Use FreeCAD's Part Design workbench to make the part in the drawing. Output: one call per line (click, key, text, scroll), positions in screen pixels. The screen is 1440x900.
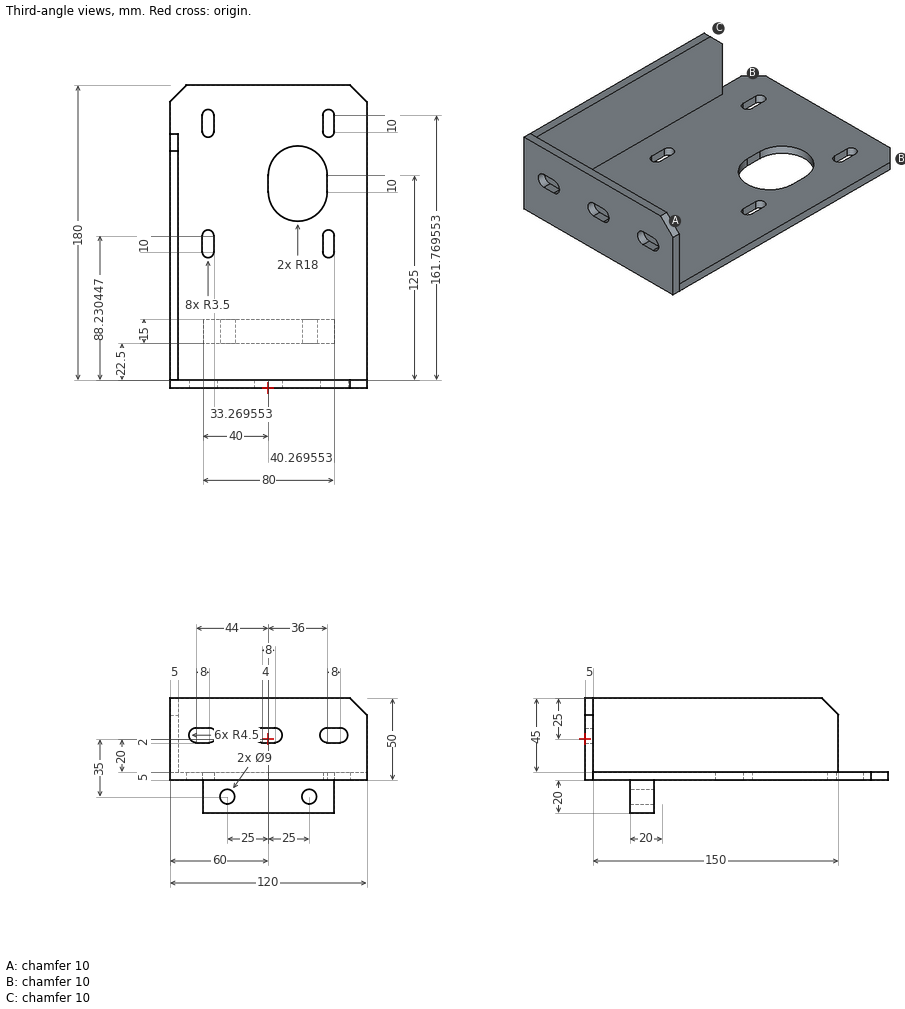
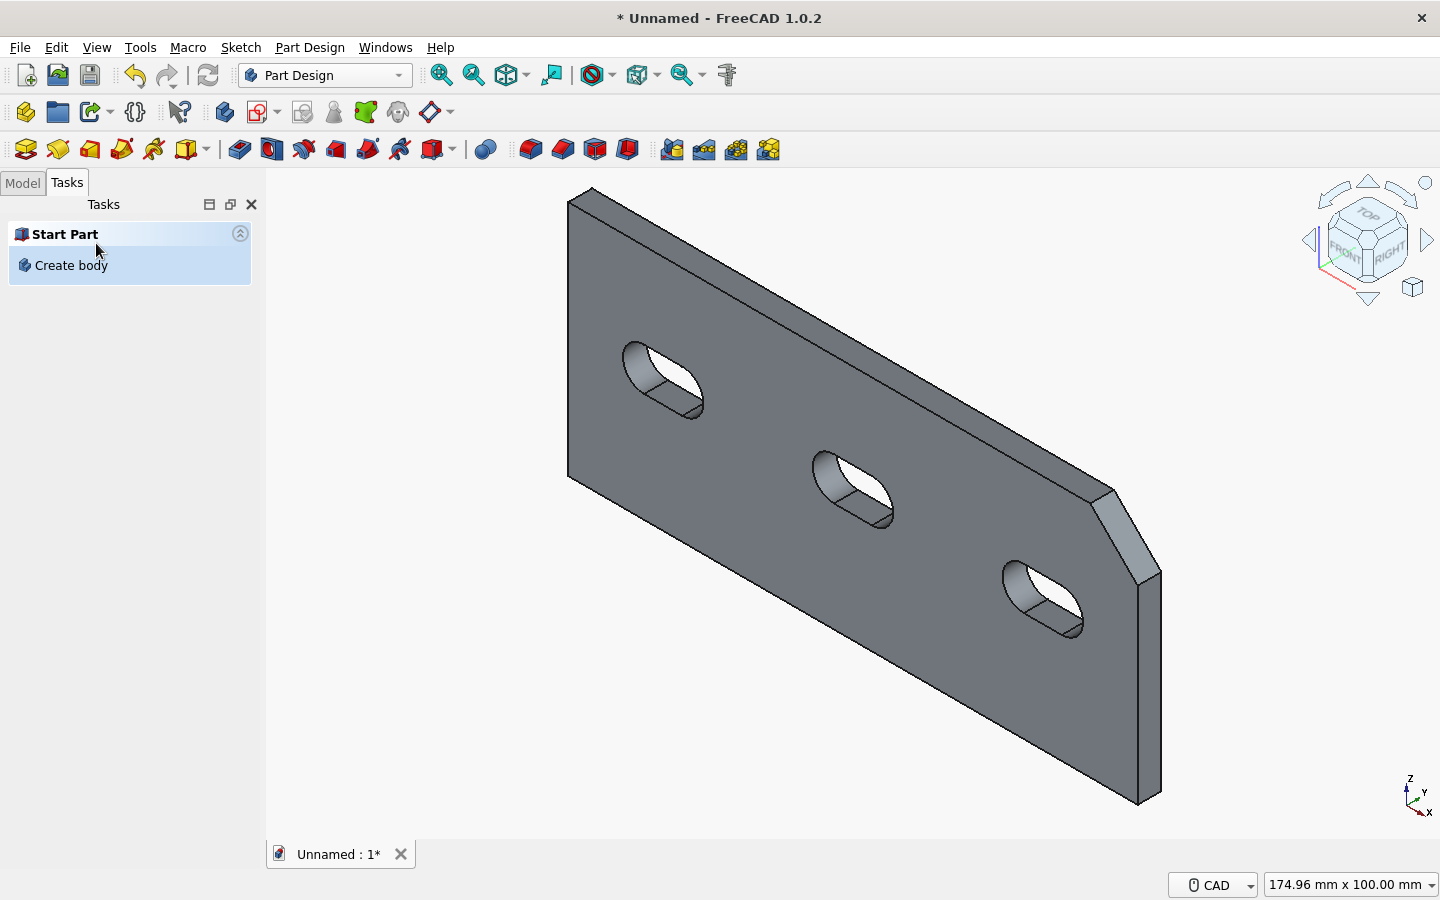
click(226, 112)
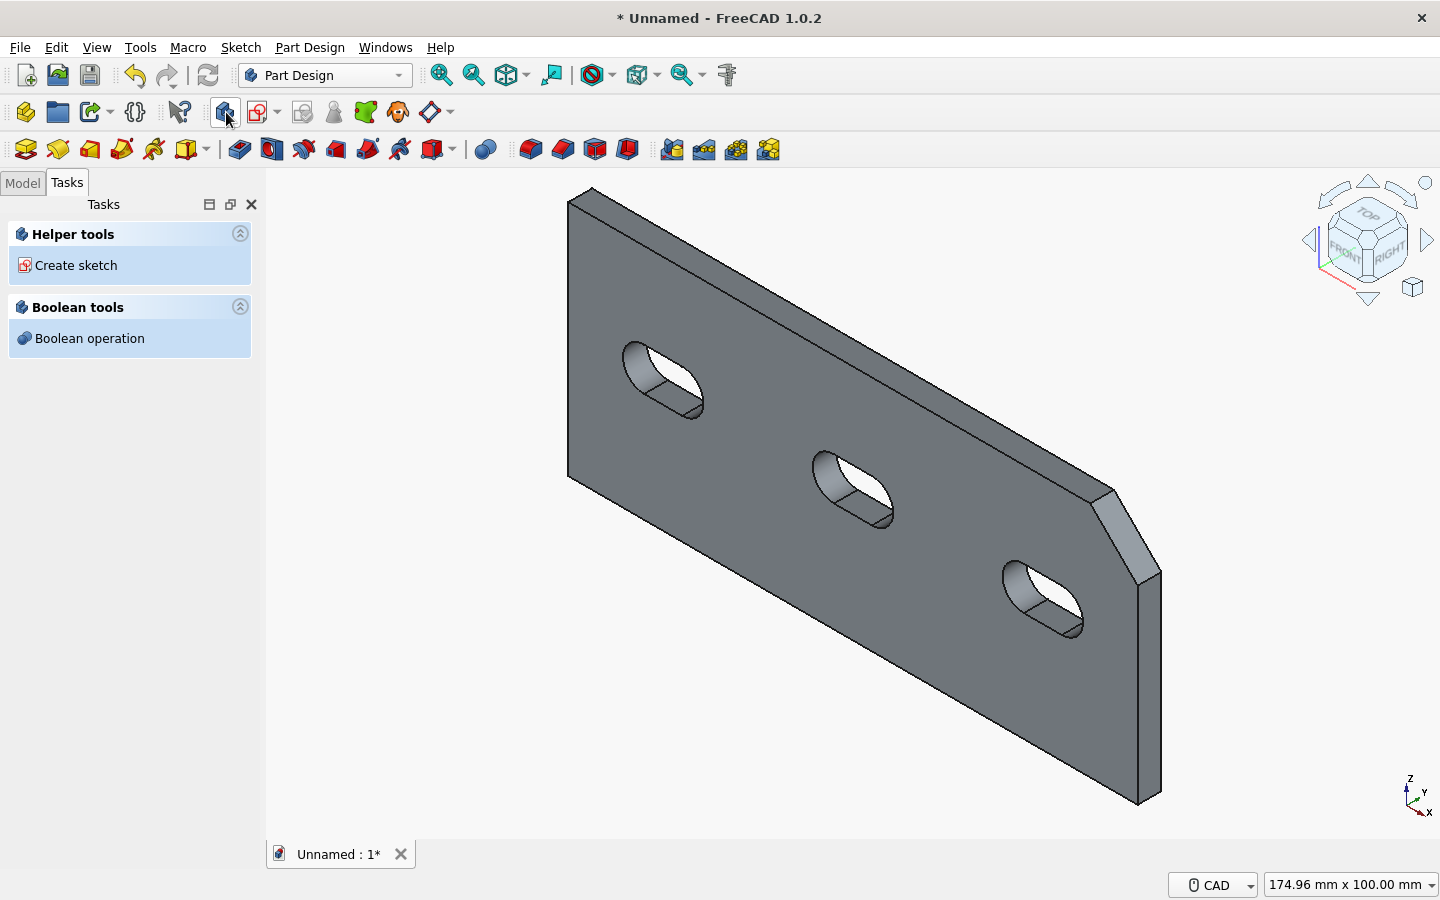
click(23, 182)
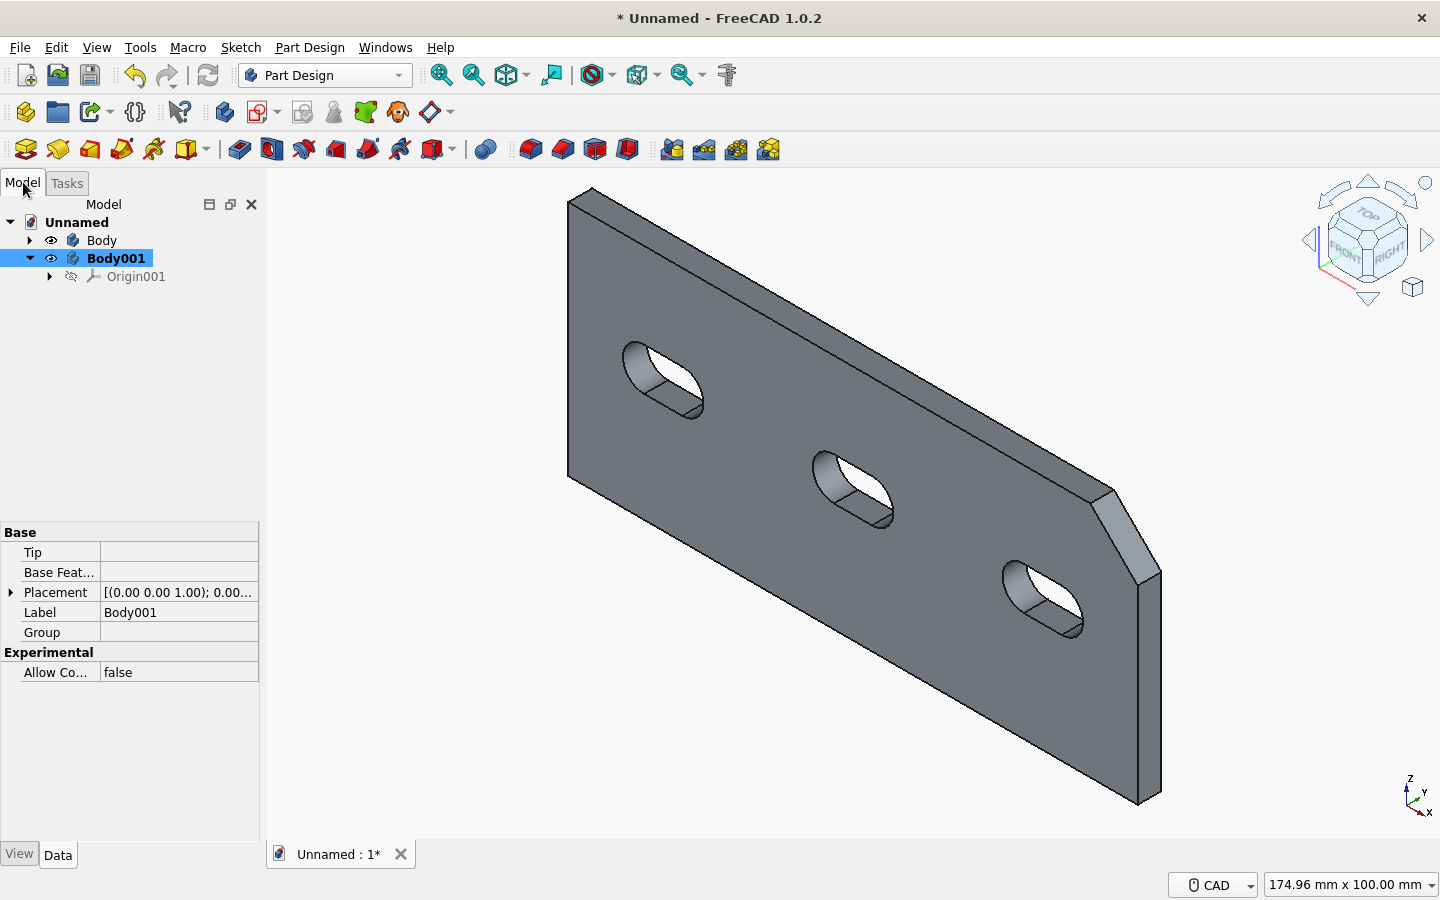
click(50, 276)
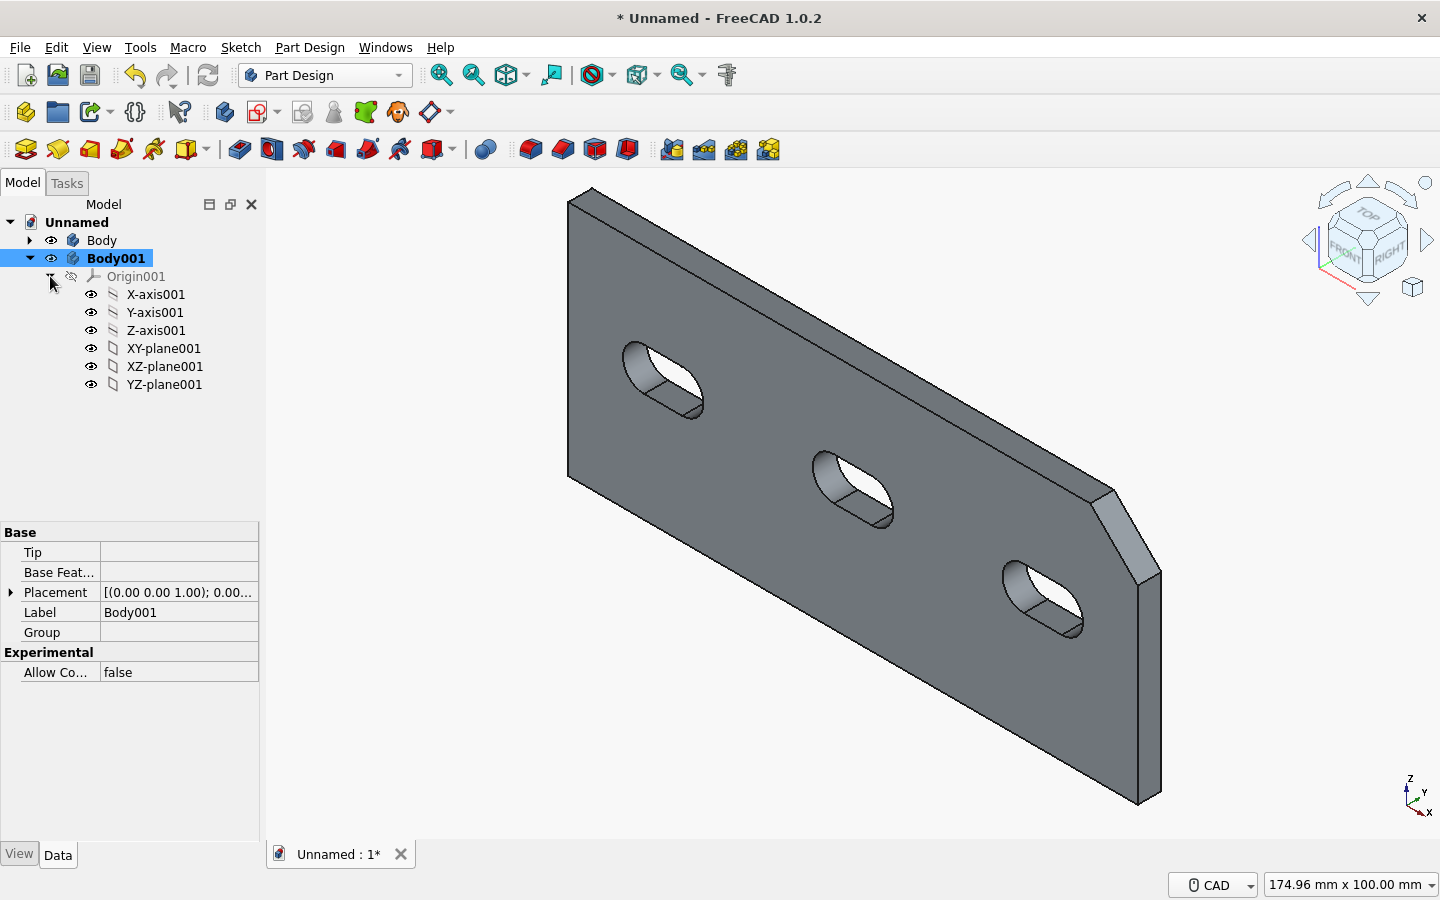
click(136, 366)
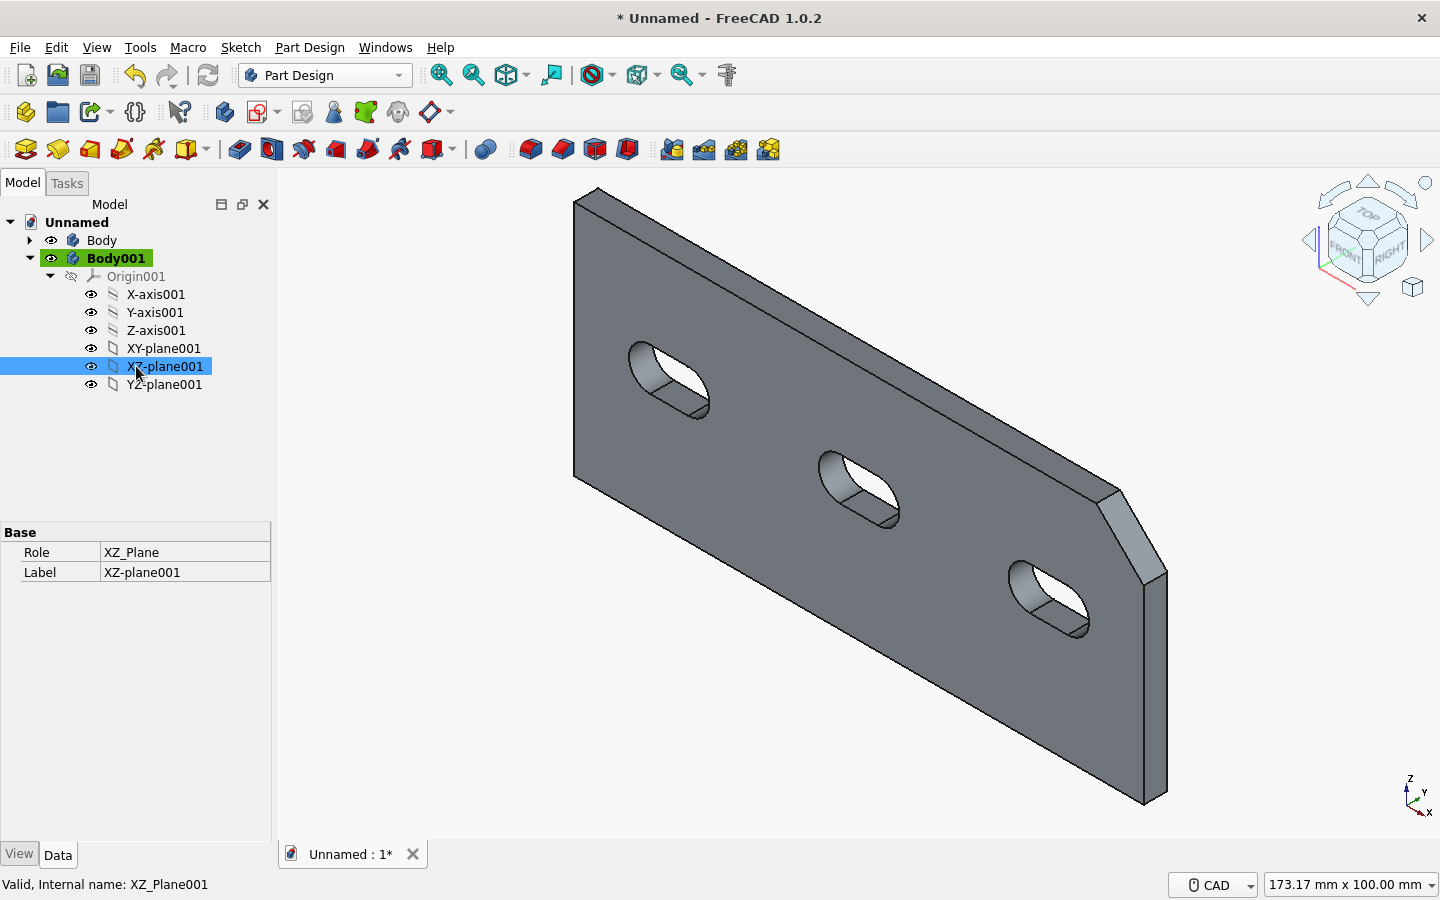
click(430, 112)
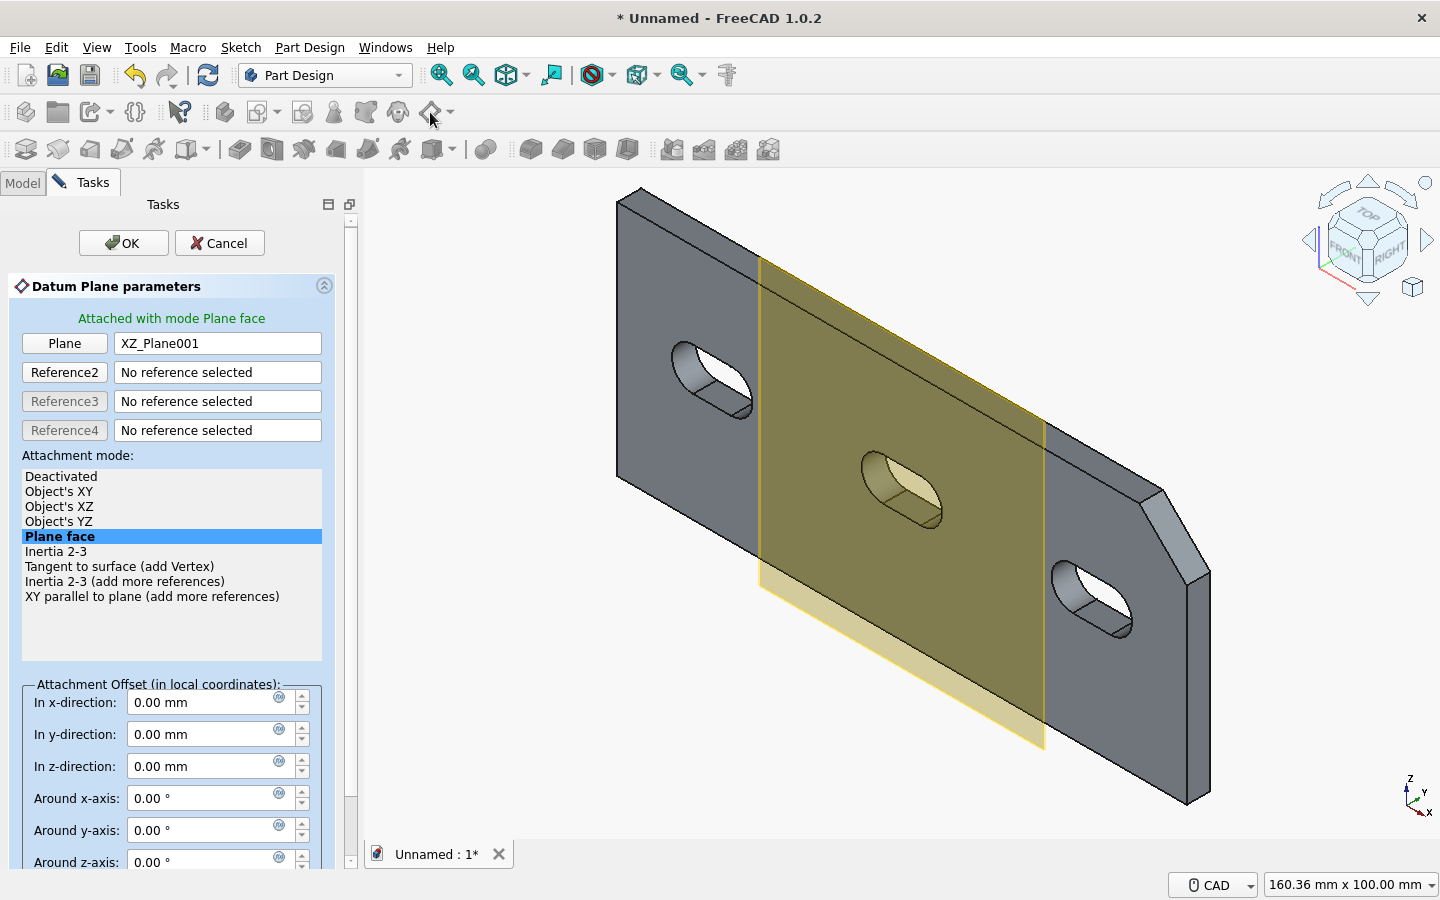
triple_click(210, 766)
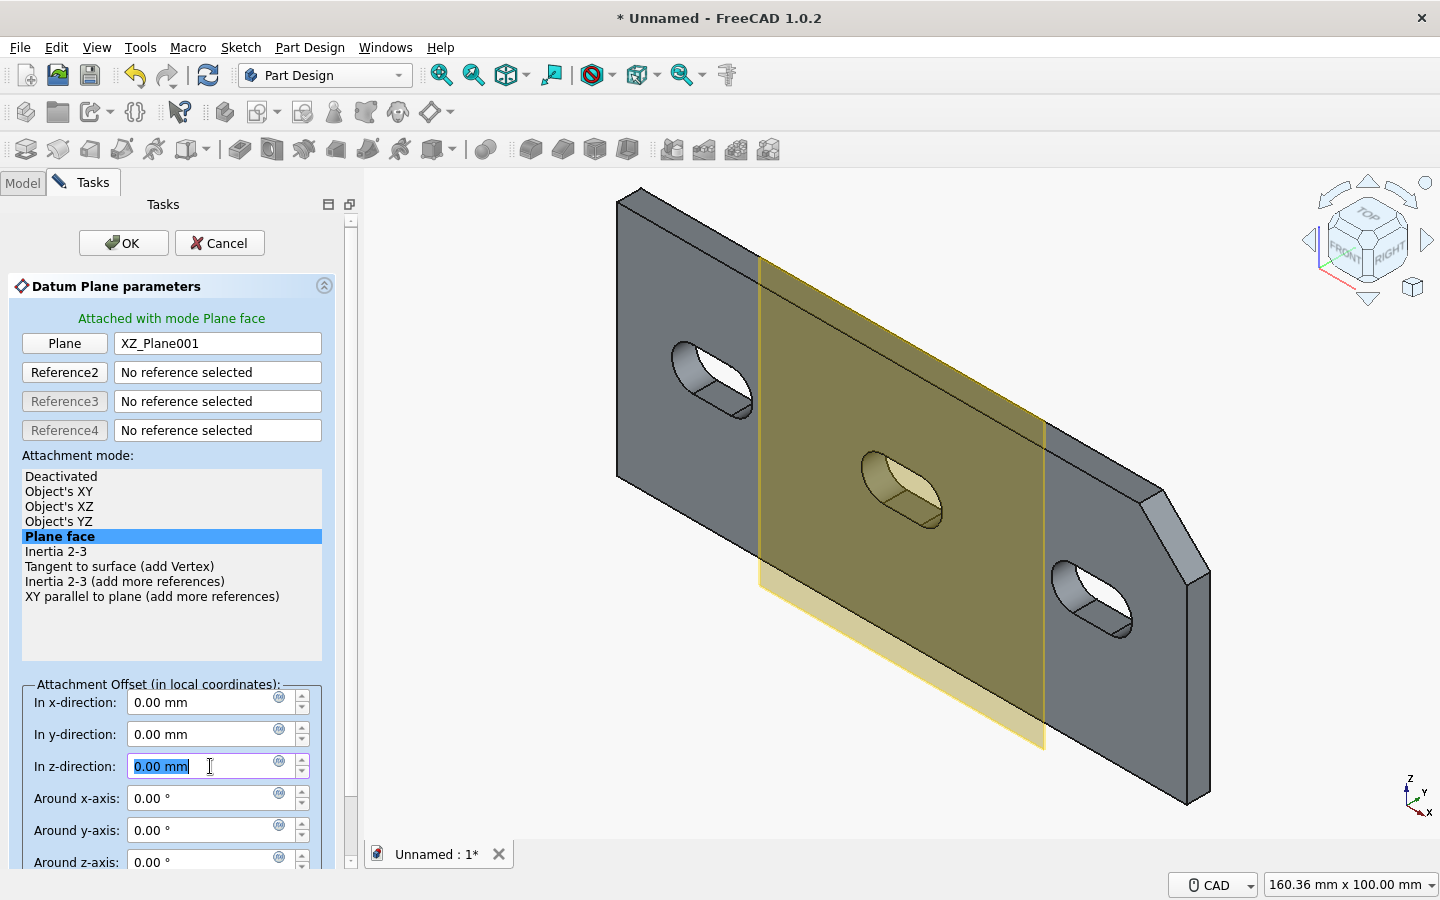
text(-5)
key(Tab)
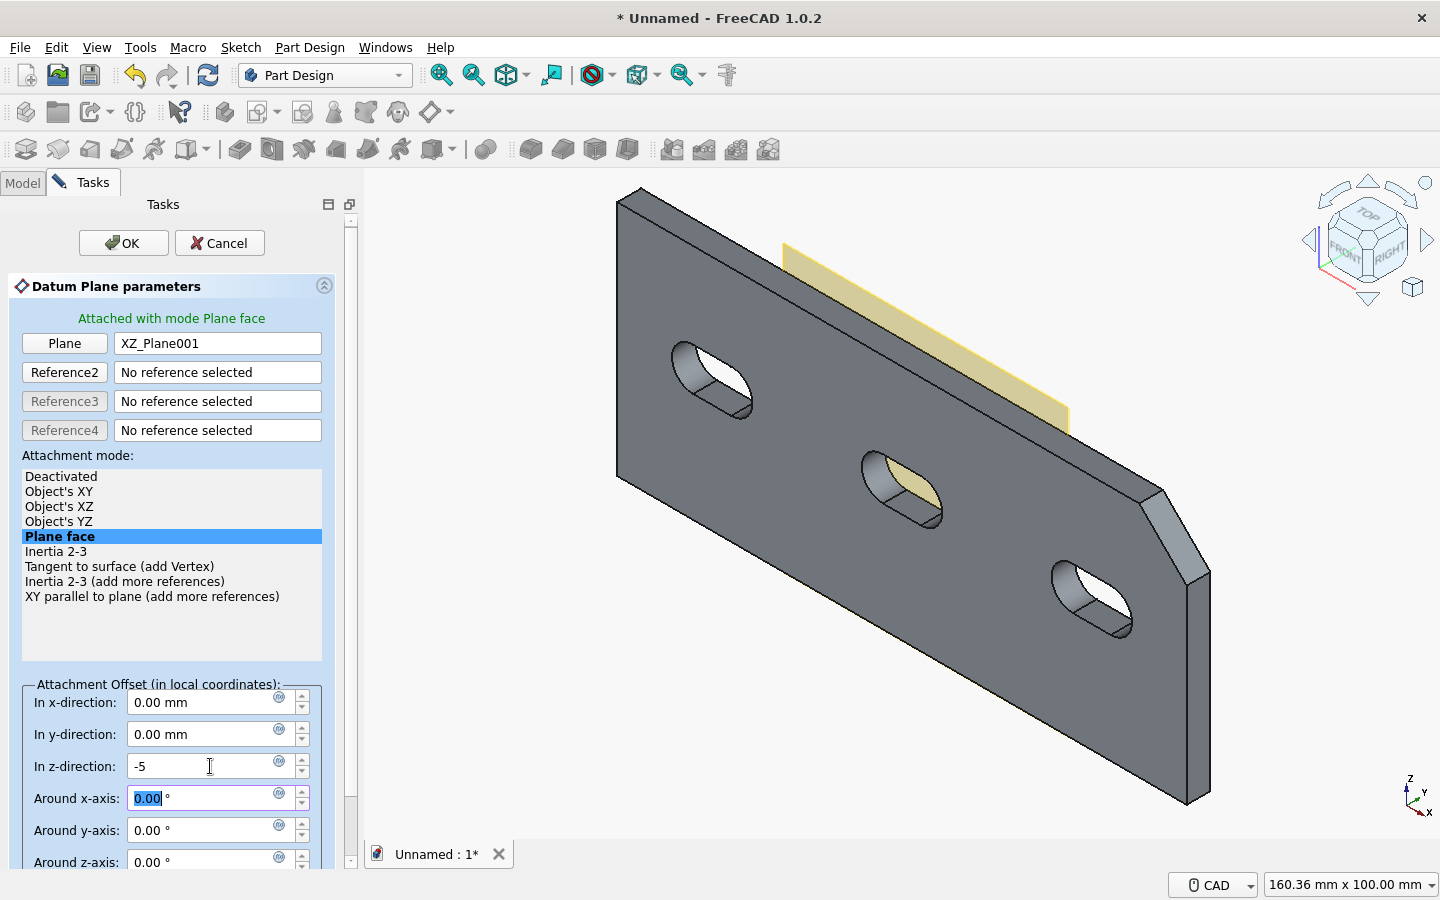
click(124, 243)